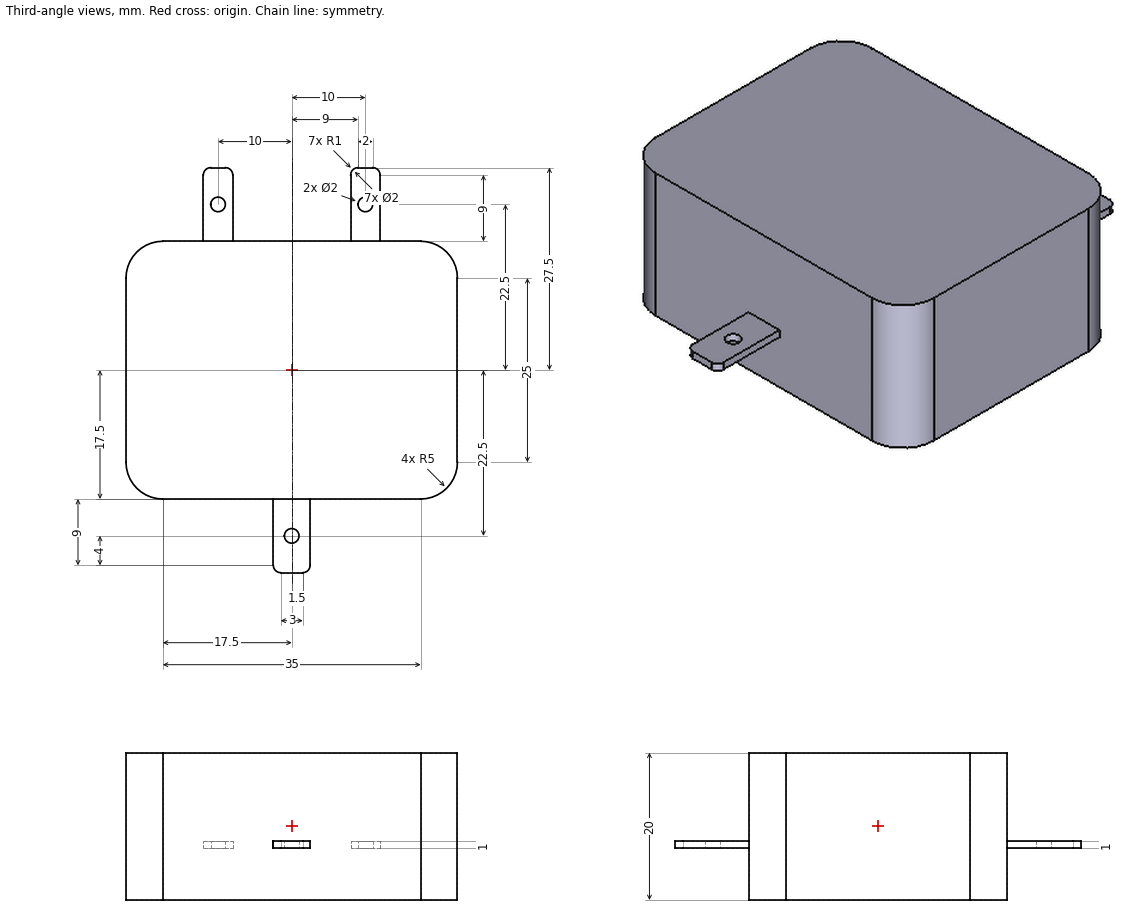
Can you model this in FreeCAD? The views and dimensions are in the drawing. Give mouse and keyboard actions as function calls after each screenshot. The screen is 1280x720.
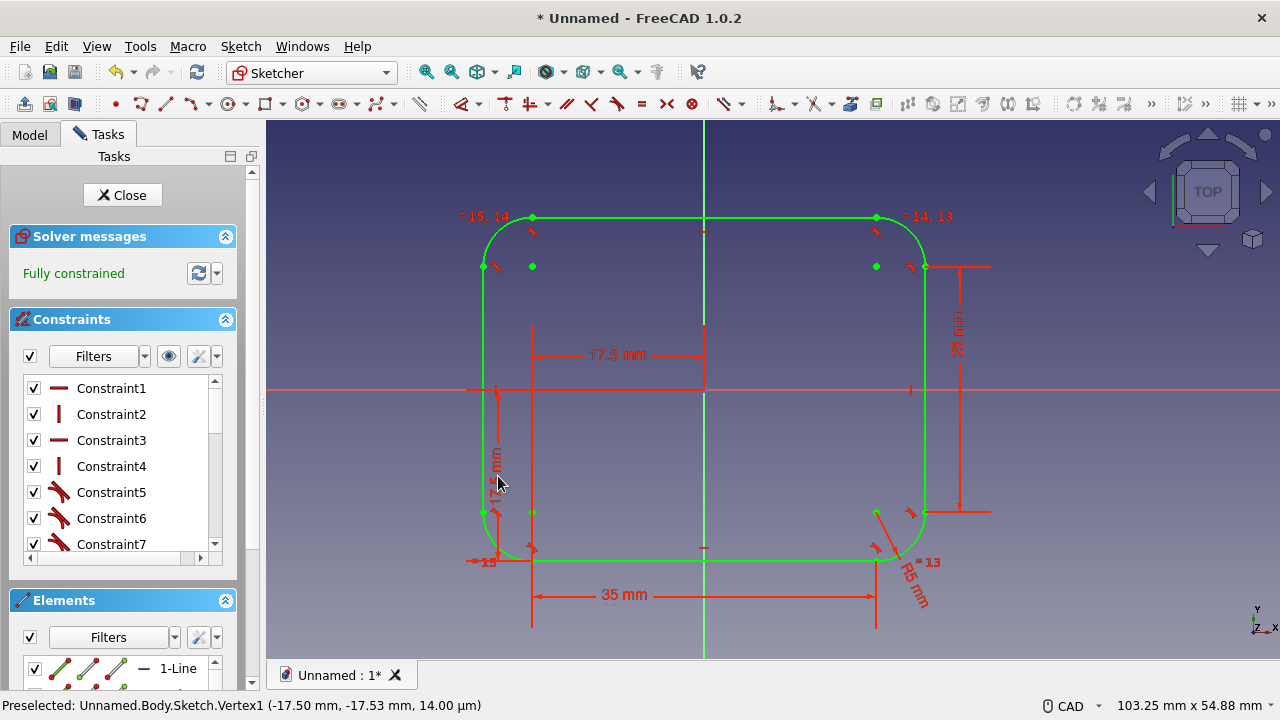
click(123, 195)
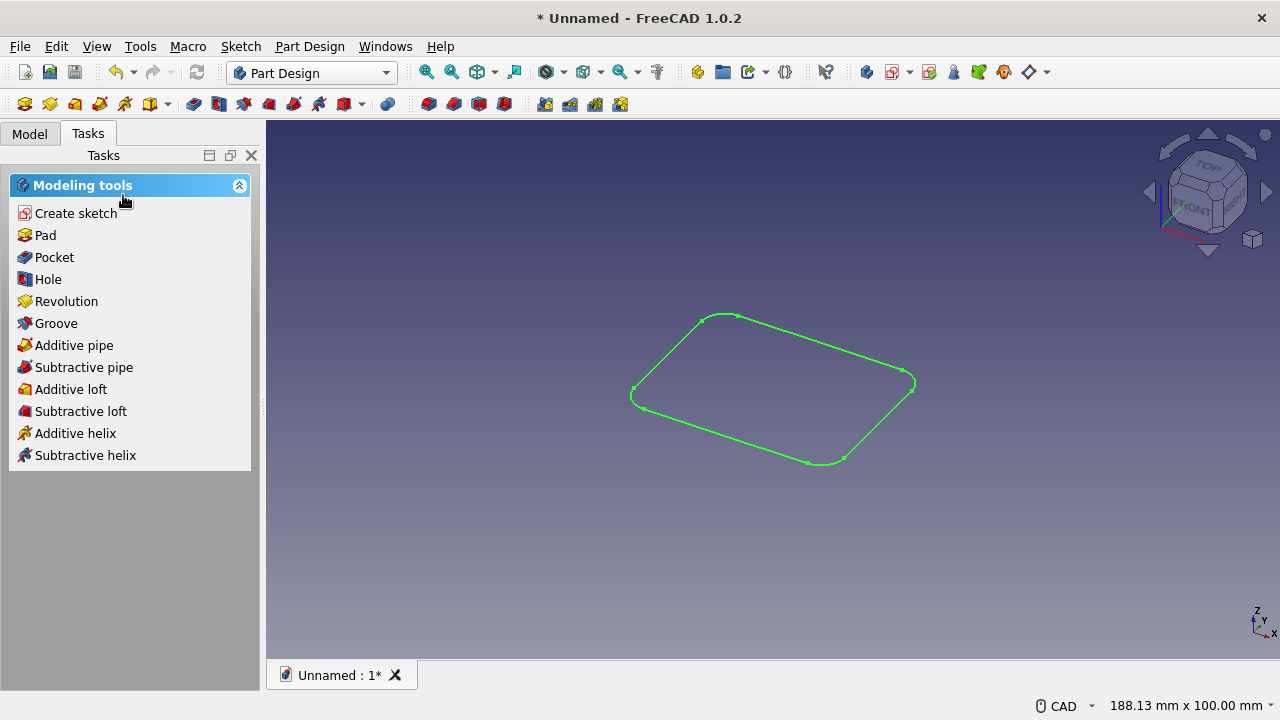
click(25, 104)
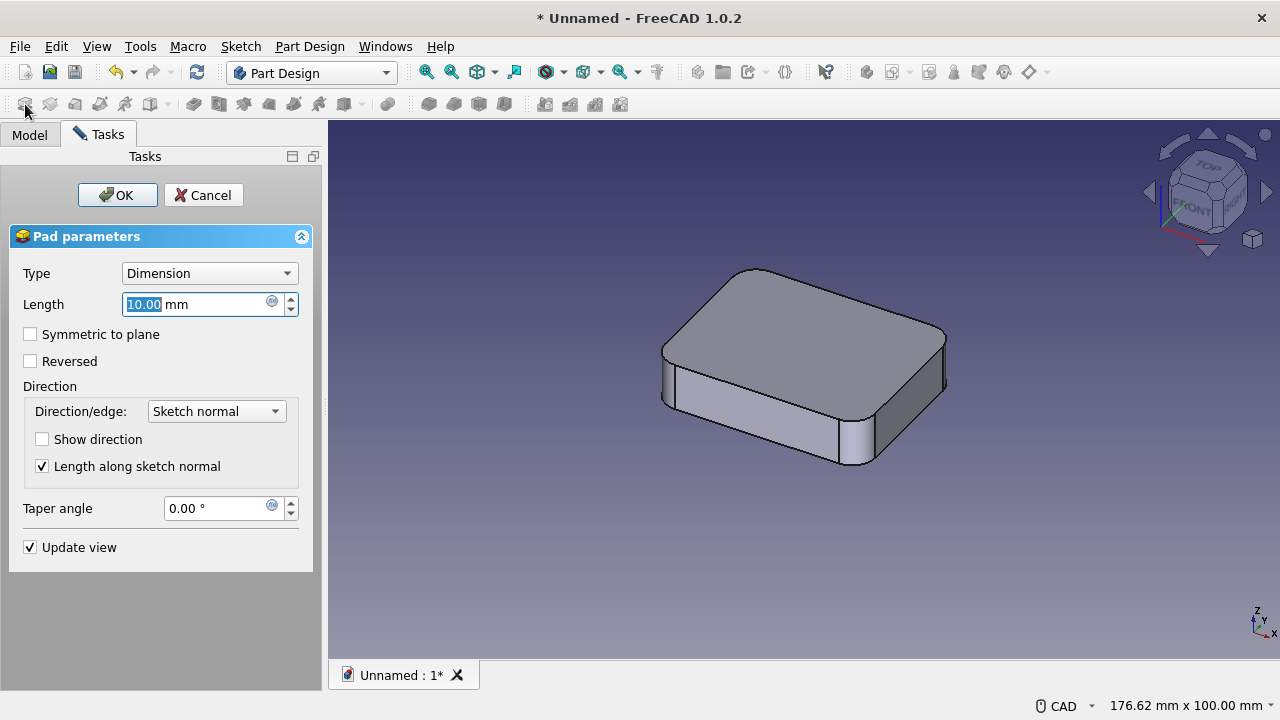
text(20)
key(Tab)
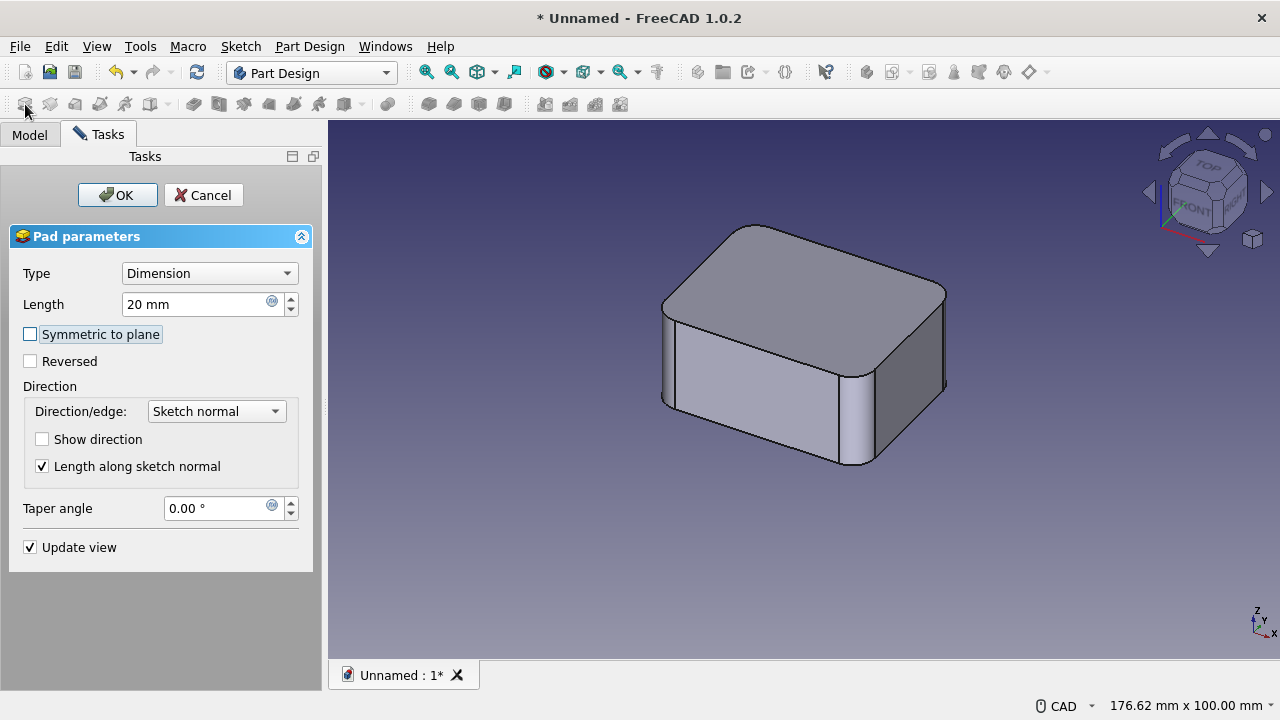
click(31, 334)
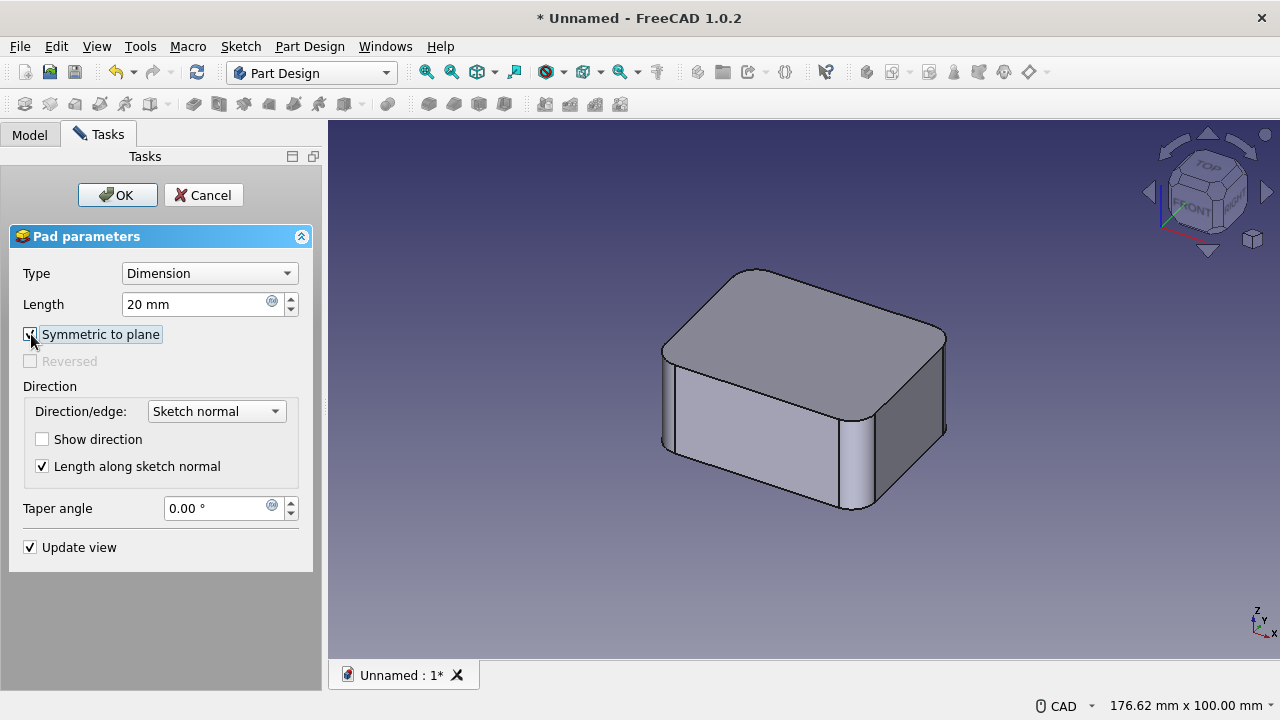
click(118, 195)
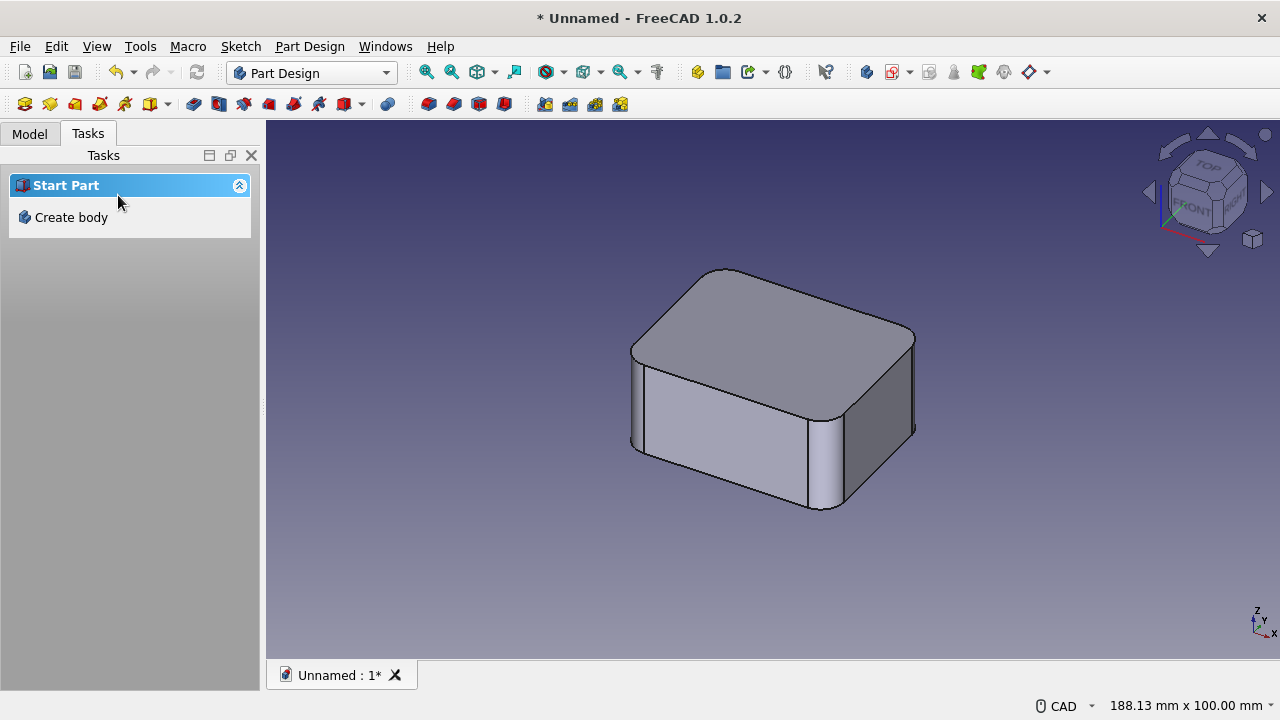
click(30, 134)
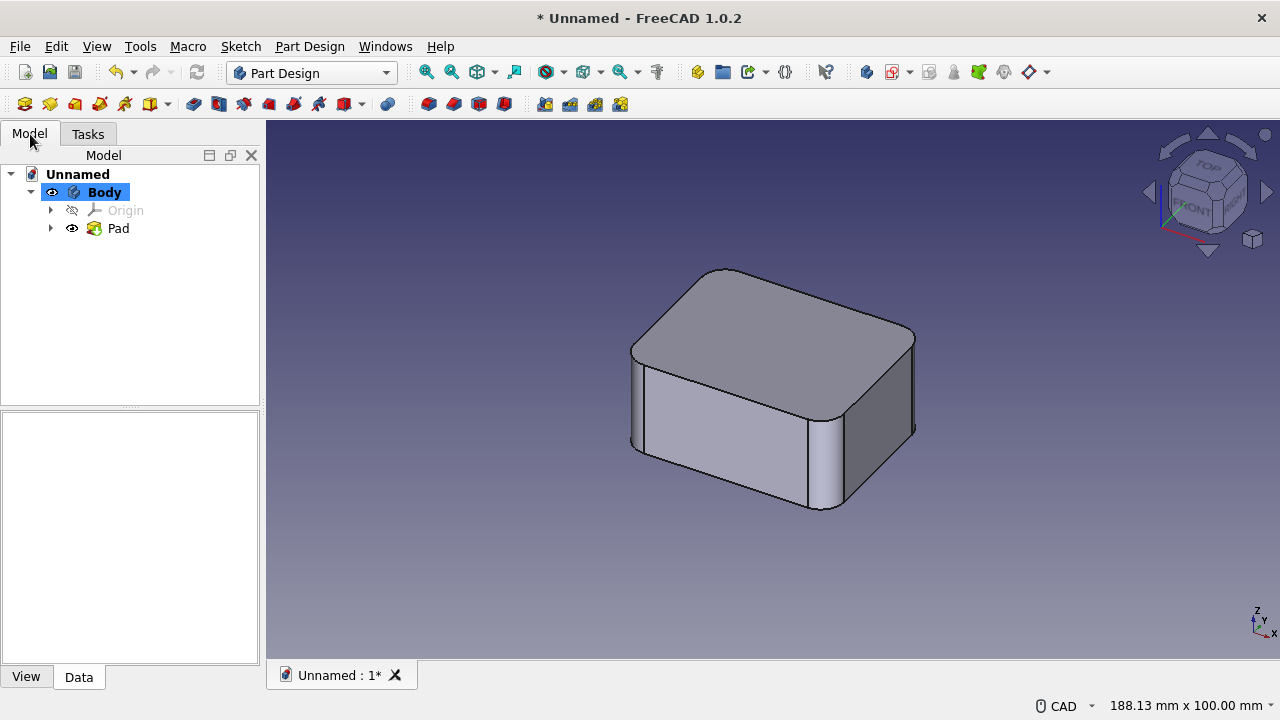
click(51, 210)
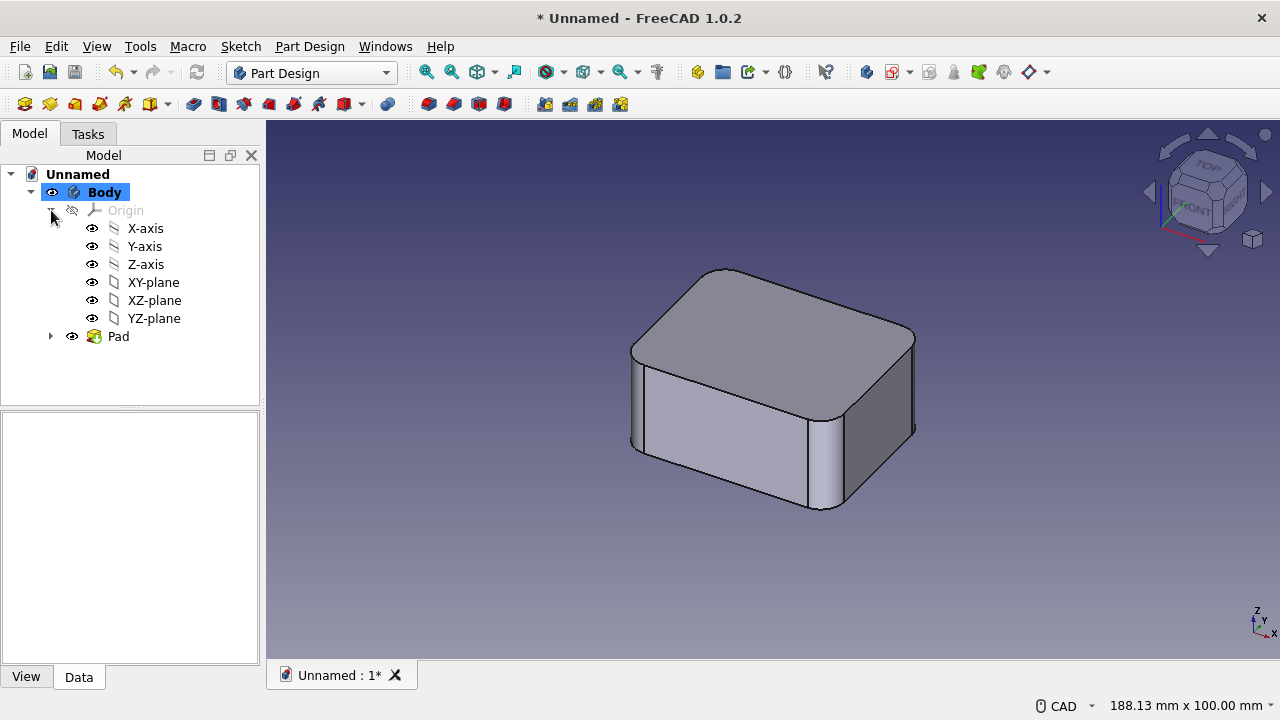
click(137, 282)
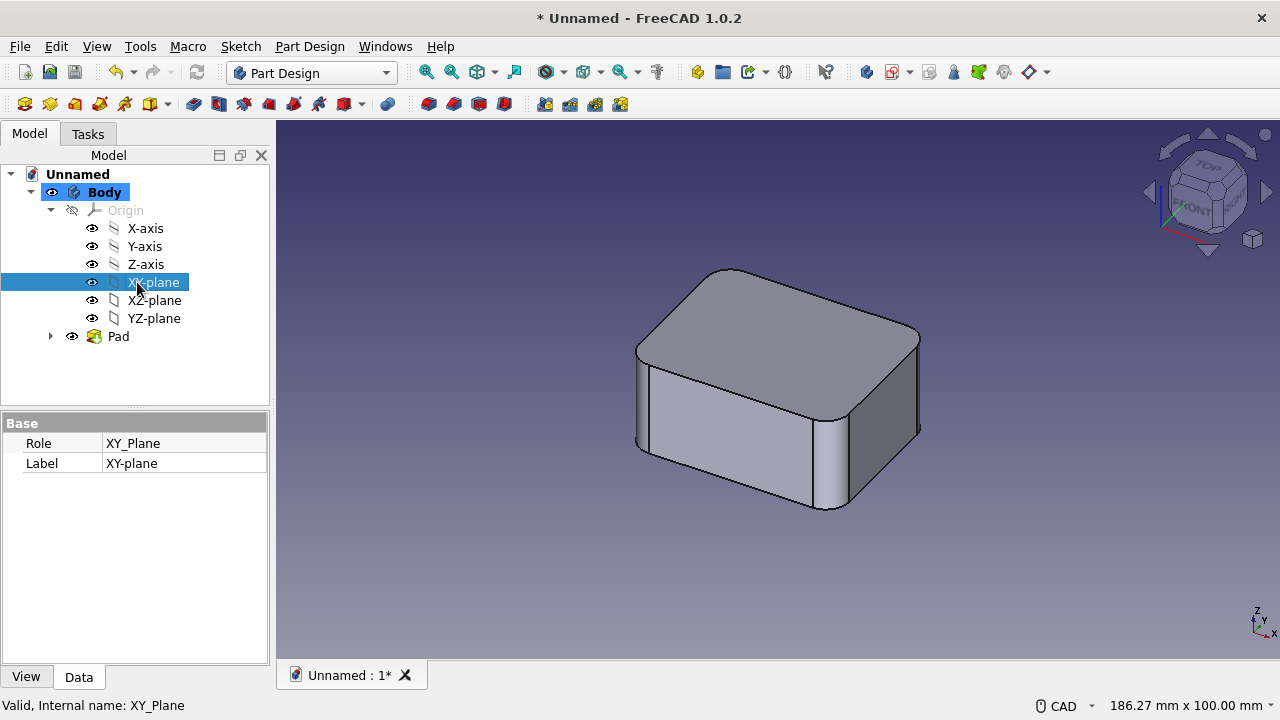
click(1028, 72)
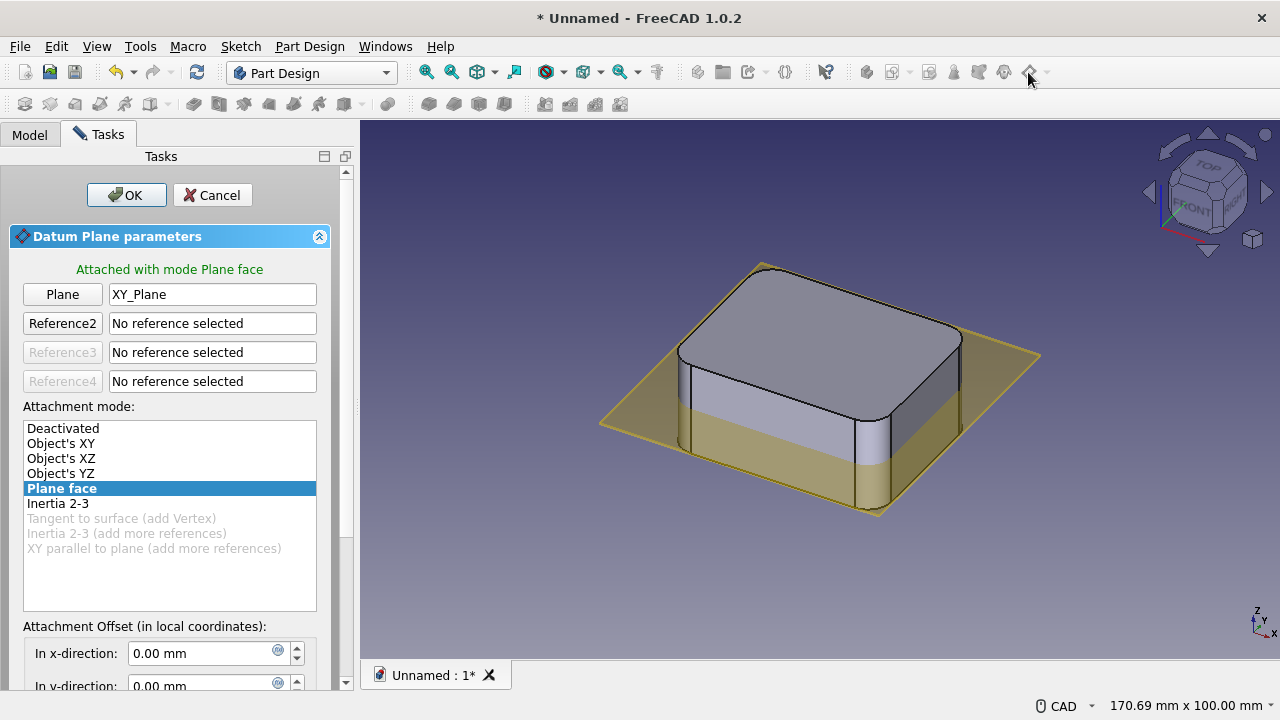
scroll(346, 428, down, 2)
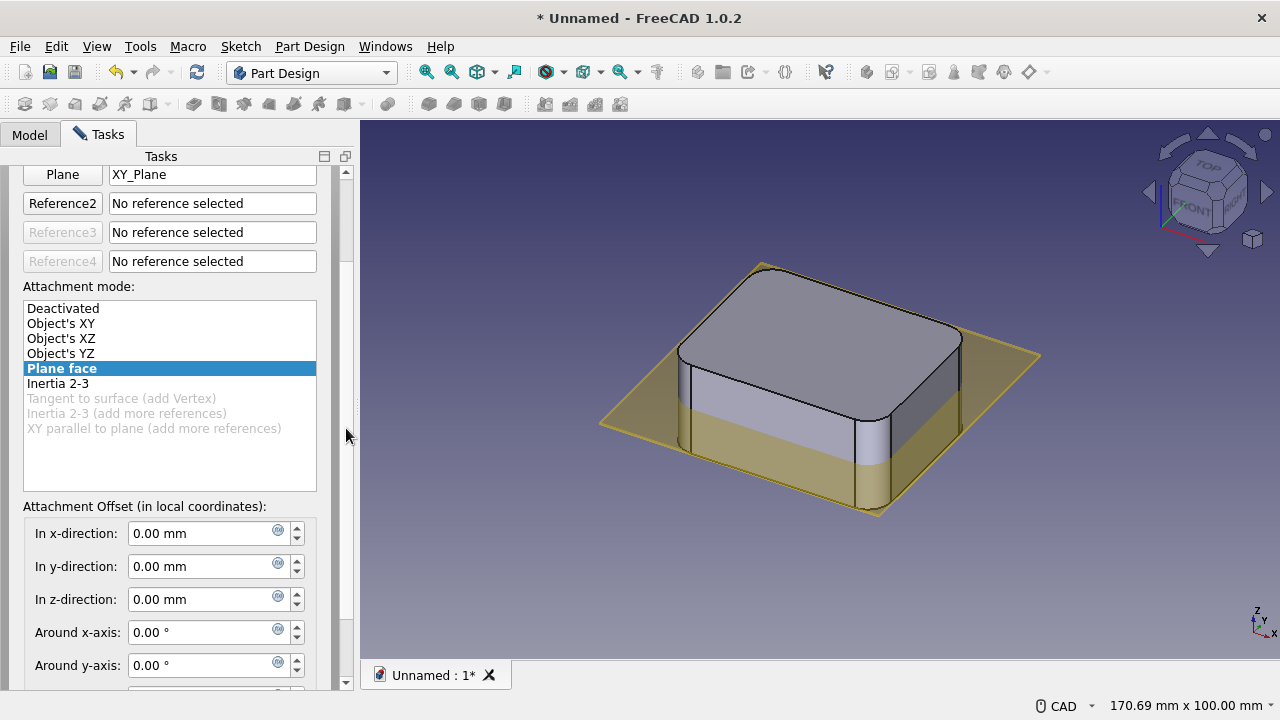
triple_click(210, 600)